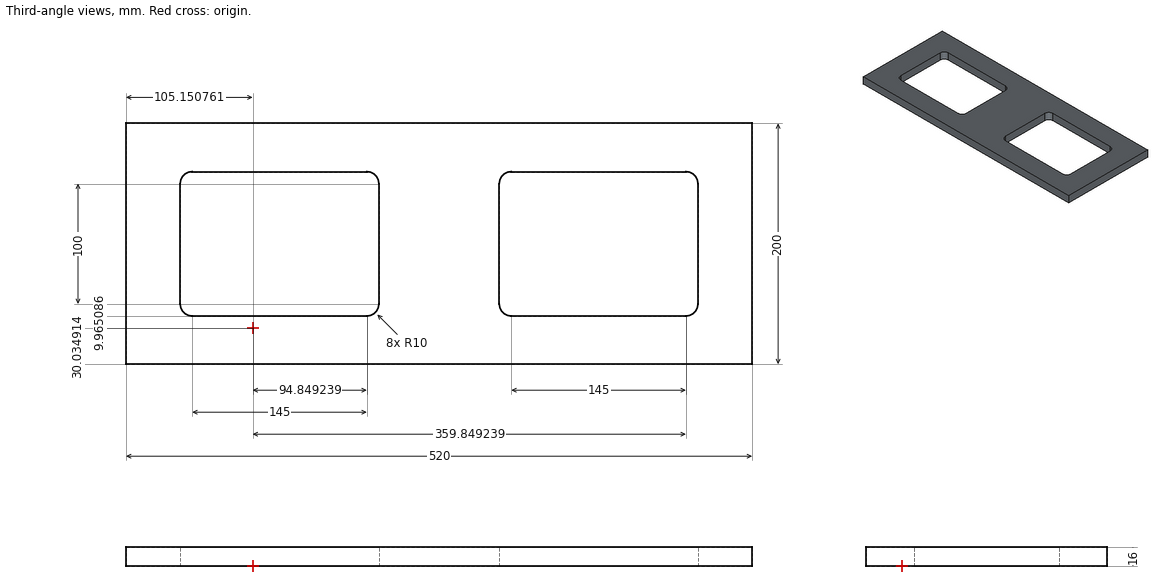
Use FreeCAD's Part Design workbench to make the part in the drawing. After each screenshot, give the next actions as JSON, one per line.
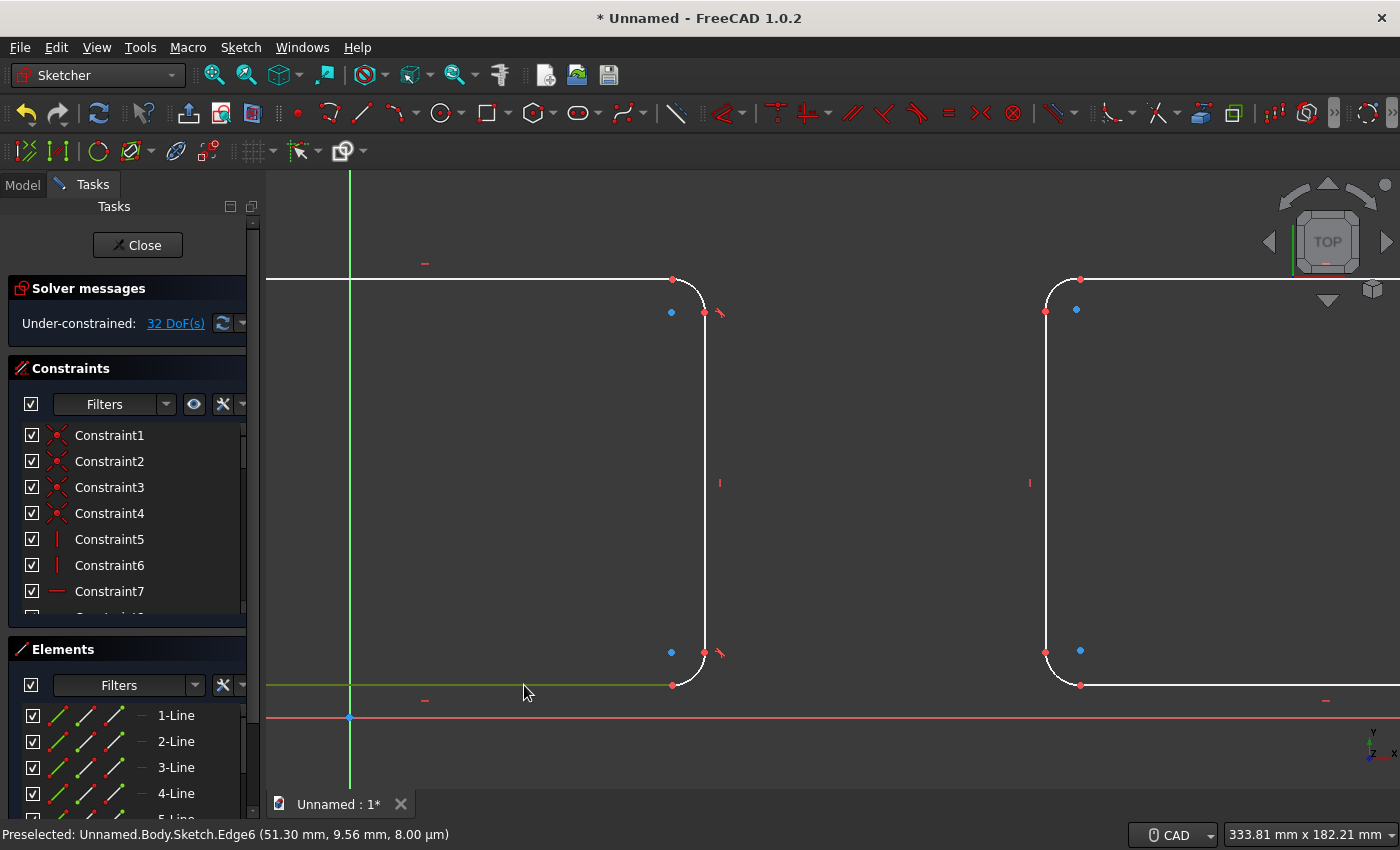
{"action": "left_click", "coordinate": [687, 682]}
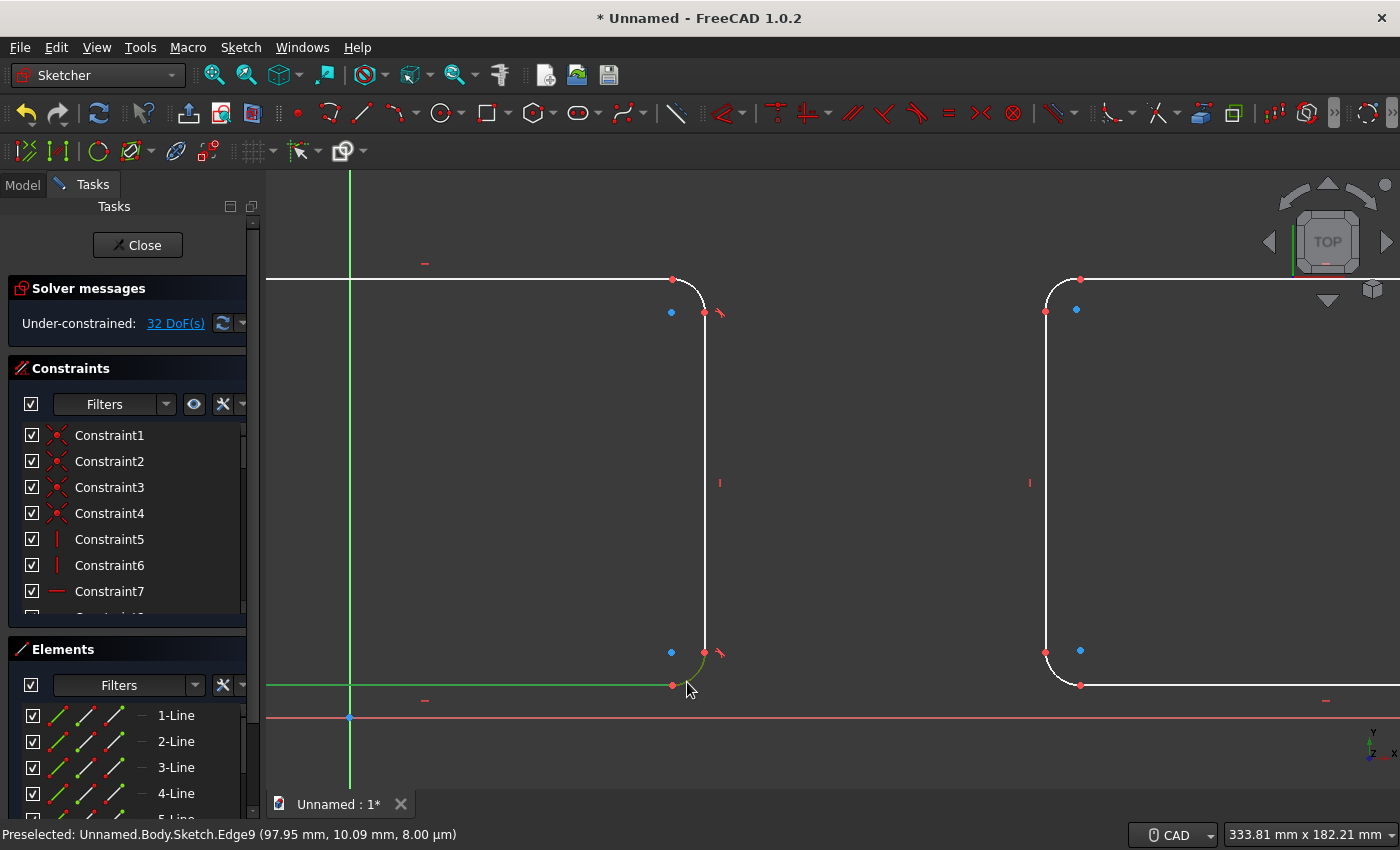
{"action": "left_click", "coordinate": [918, 114]}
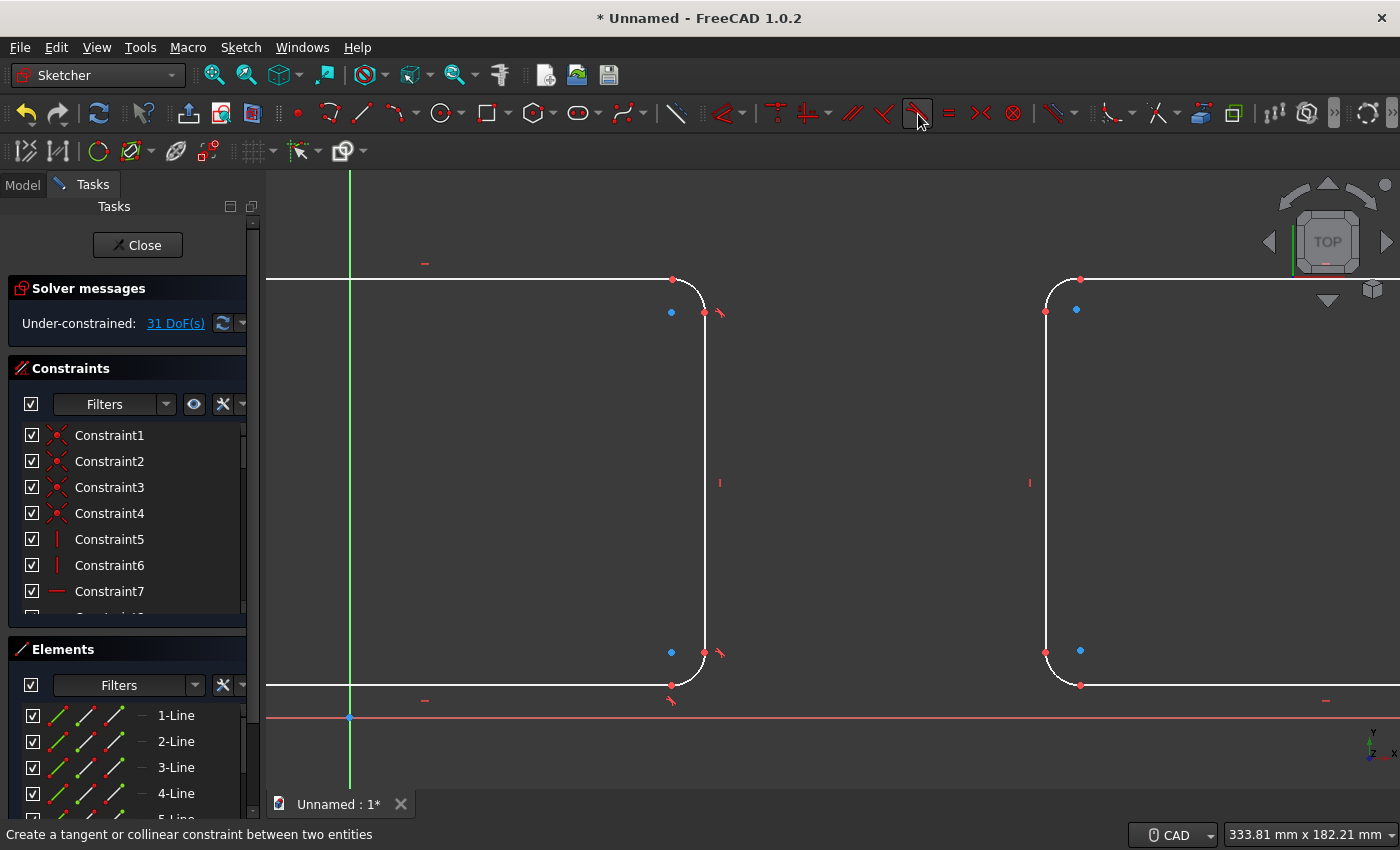
{"action": "left_click", "coordinate": [524, 685]}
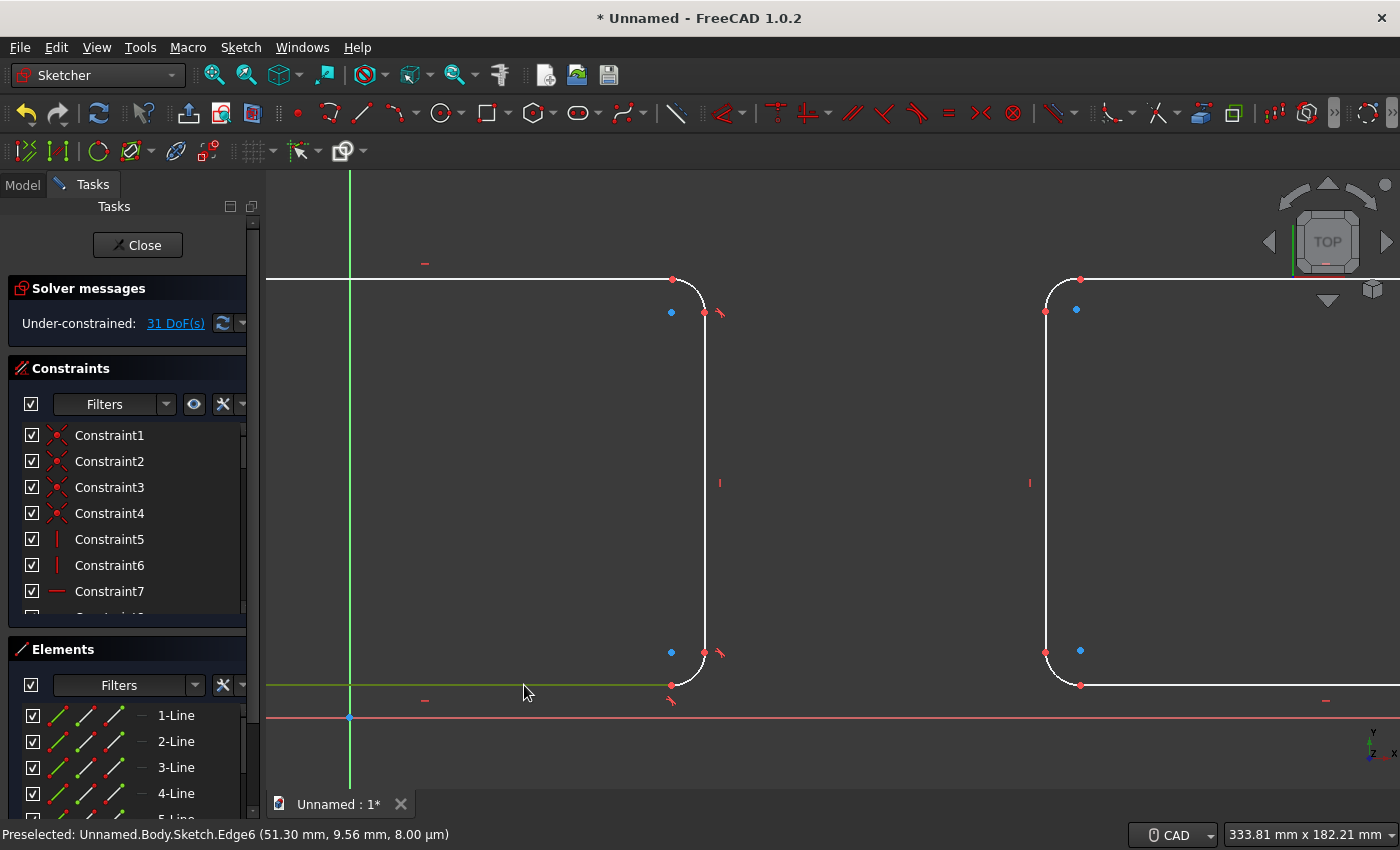
{"action": "scroll", "coordinate": [700, 479], "scroll_direction": "down", "scroll_amount": 5}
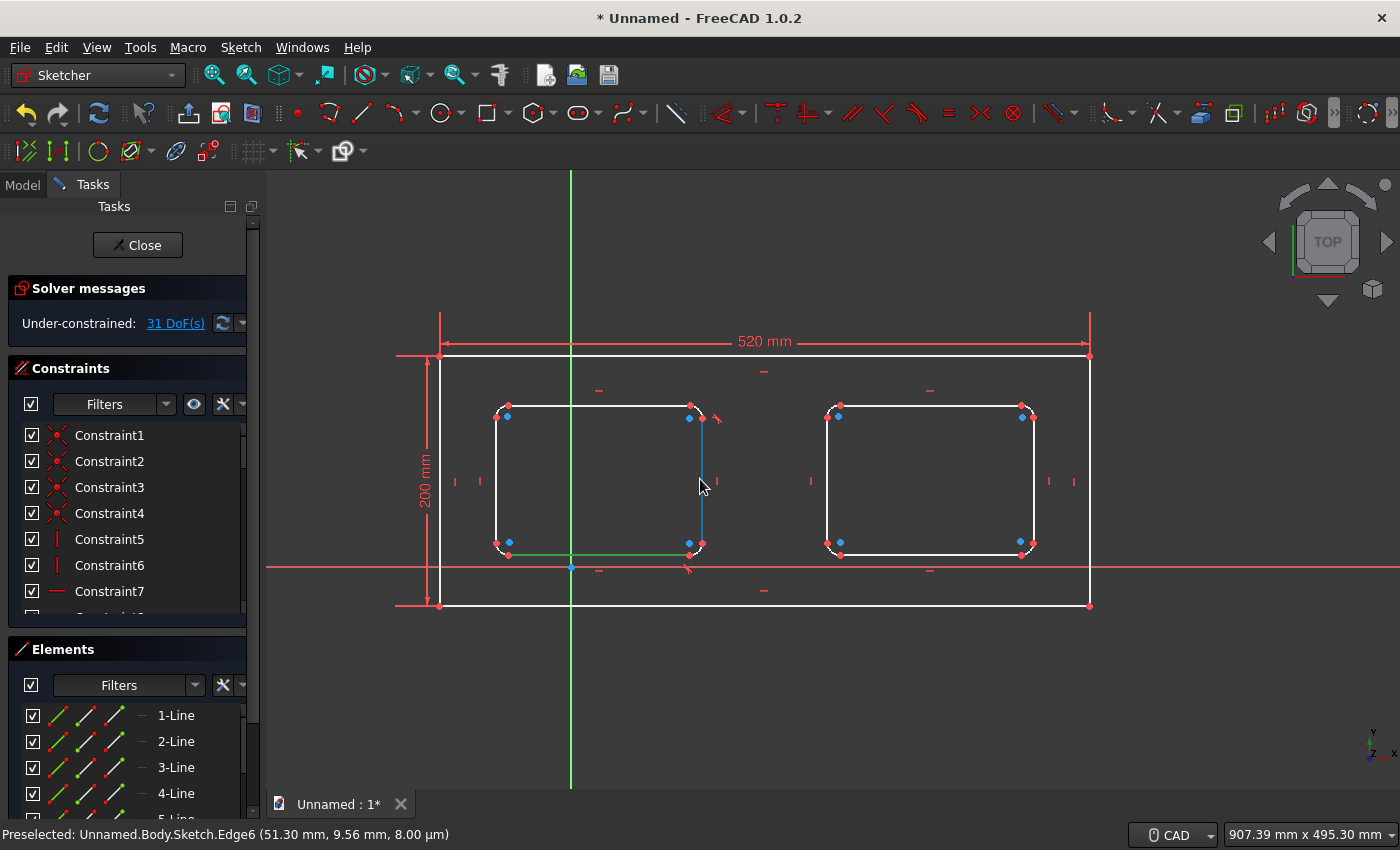
{"action": "scroll", "coordinate": [498, 549], "scroll_direction": "up", "scroll_amount": 5}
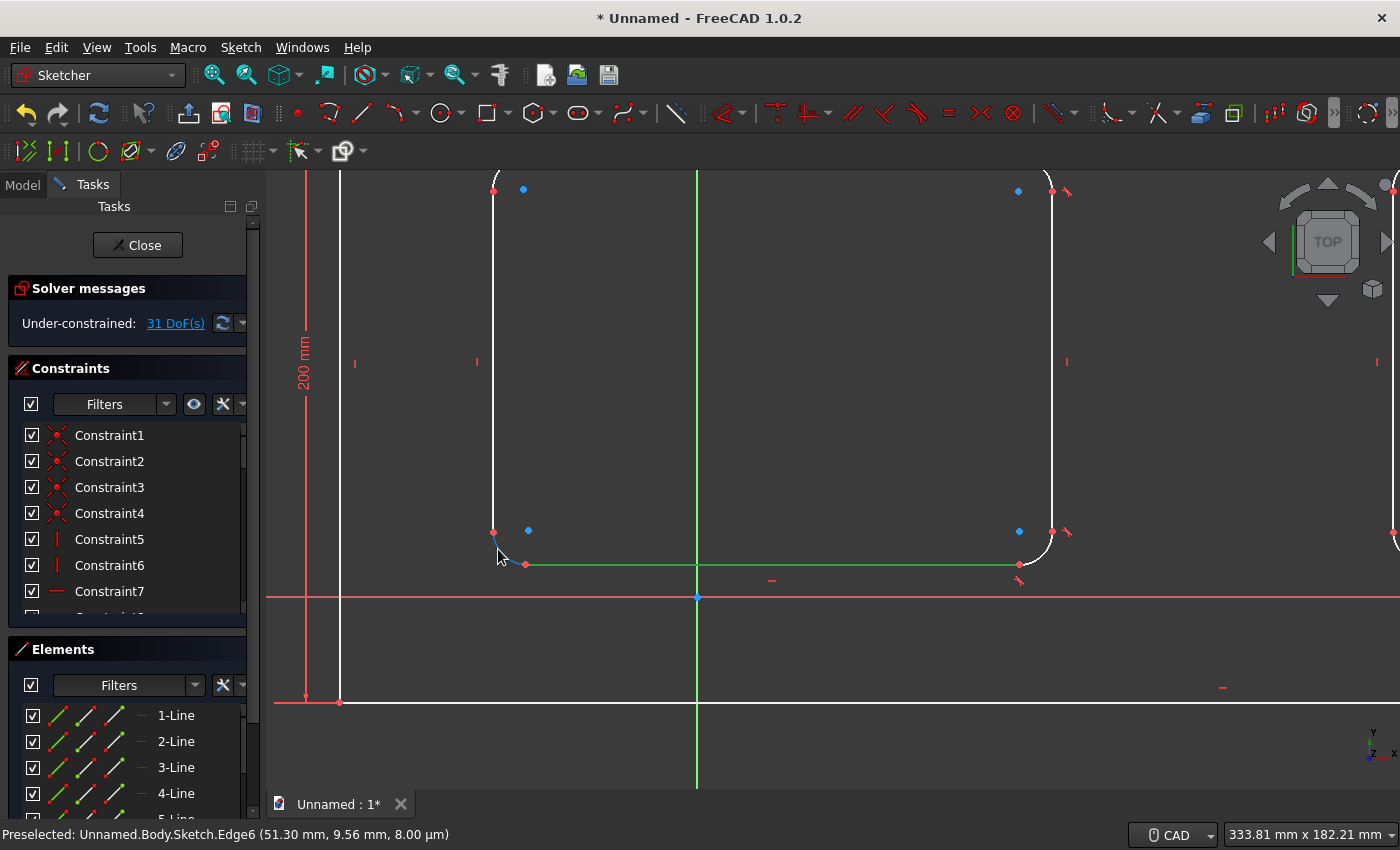
{"action": "left_click", "coordinate": [497, 547]}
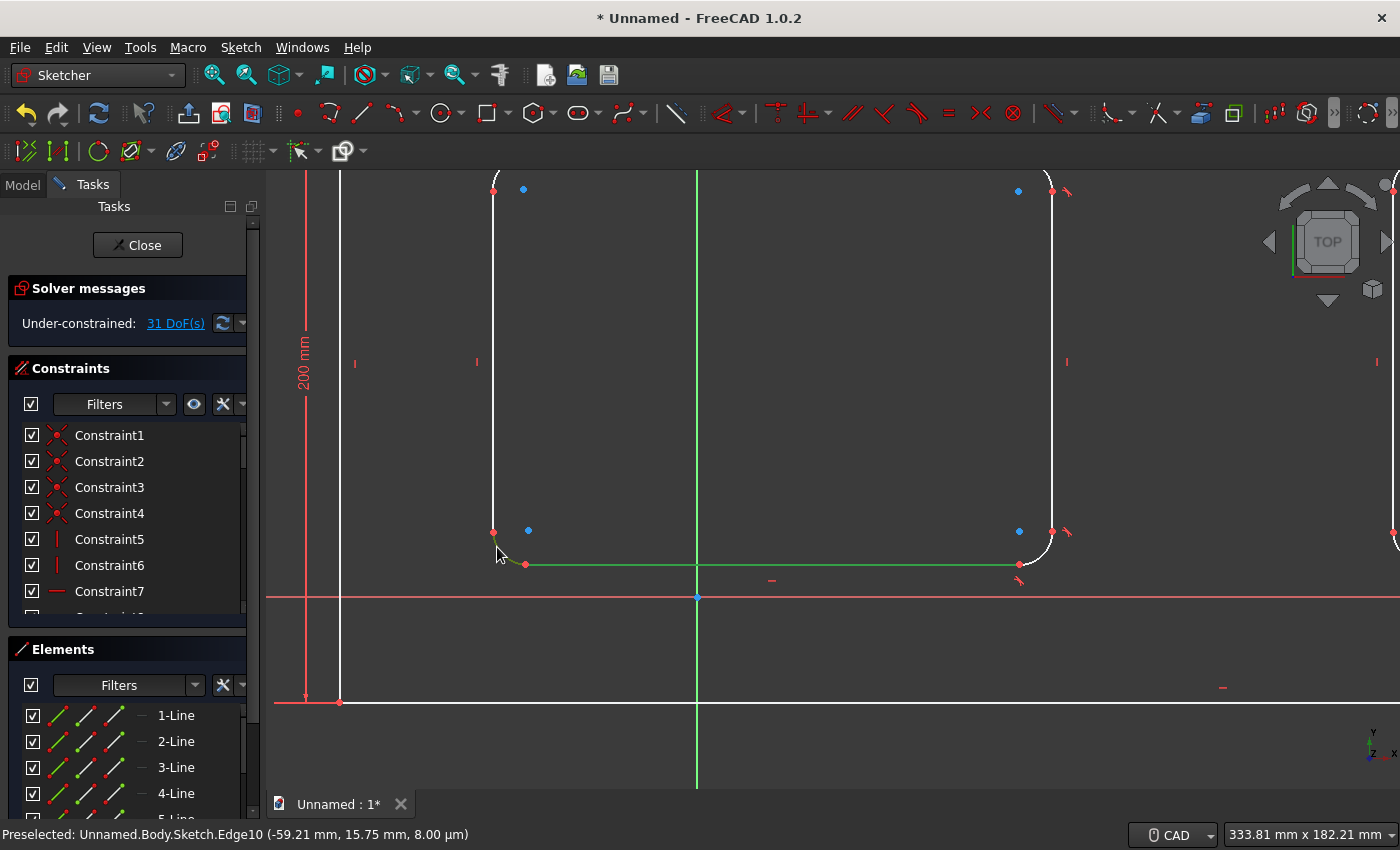
{"action": "key", "text": "t"}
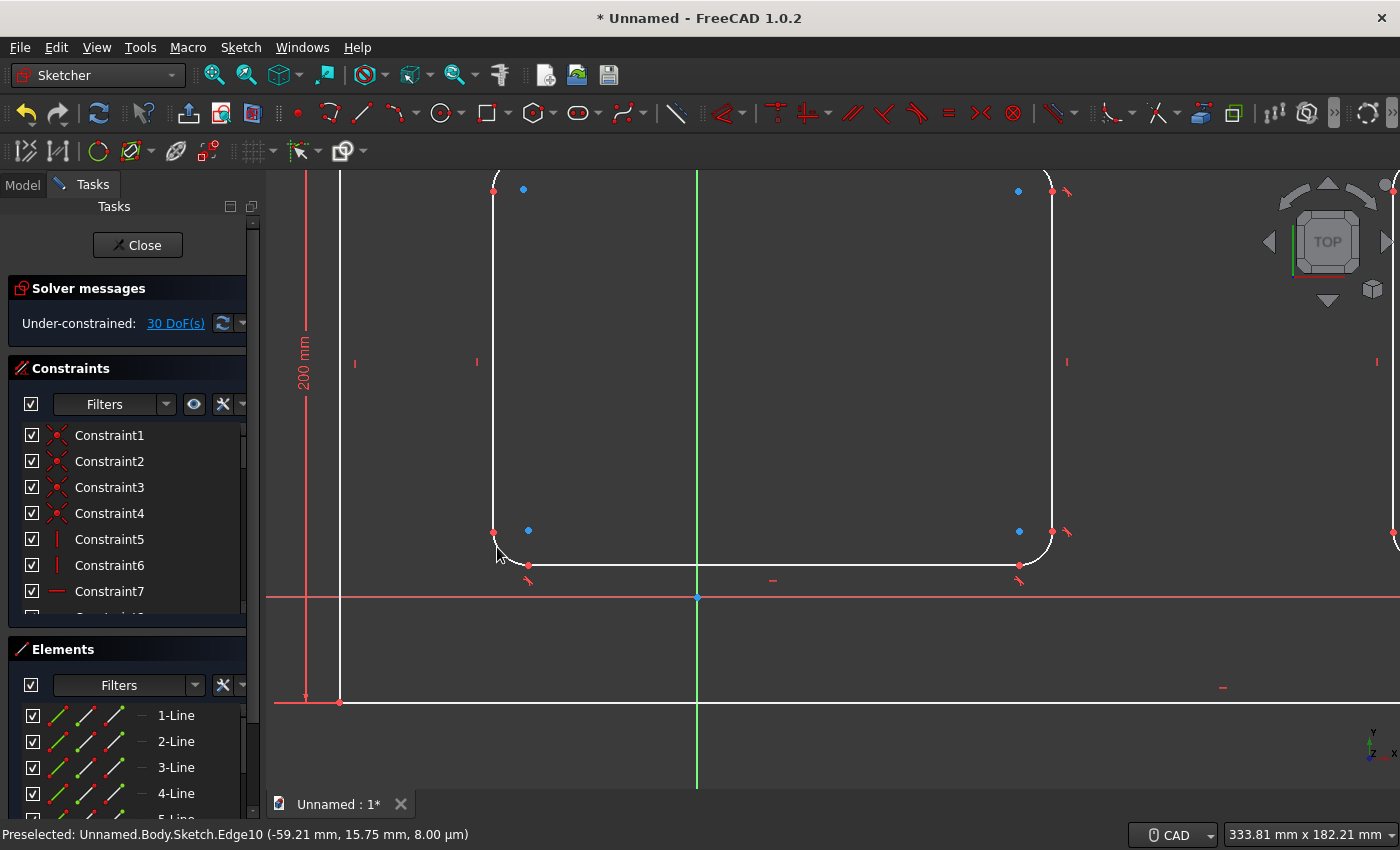
{"action": "left_click", "coordinate": [493, 430]}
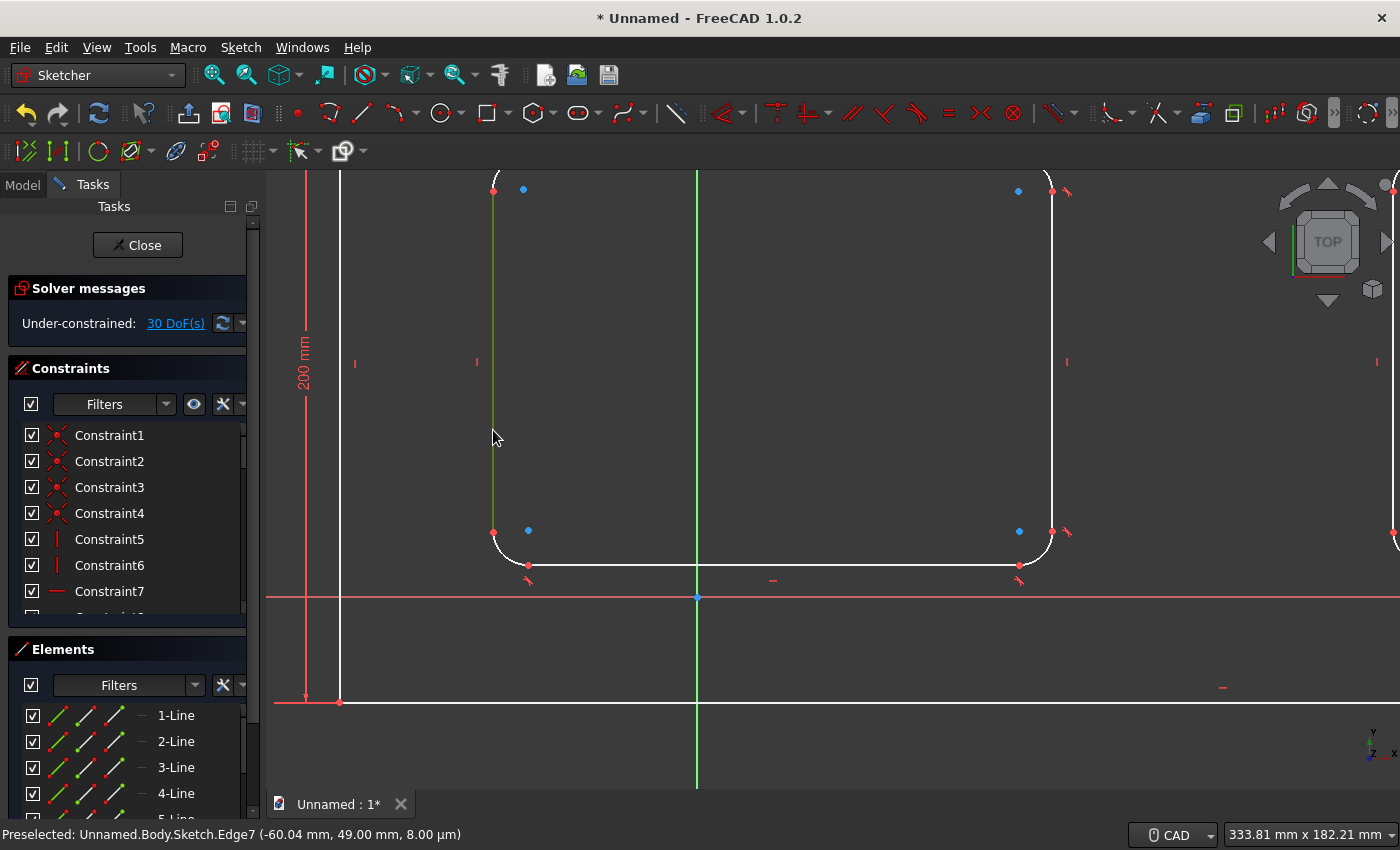
{"action": "left_click", "coordinate": [498, 547]}